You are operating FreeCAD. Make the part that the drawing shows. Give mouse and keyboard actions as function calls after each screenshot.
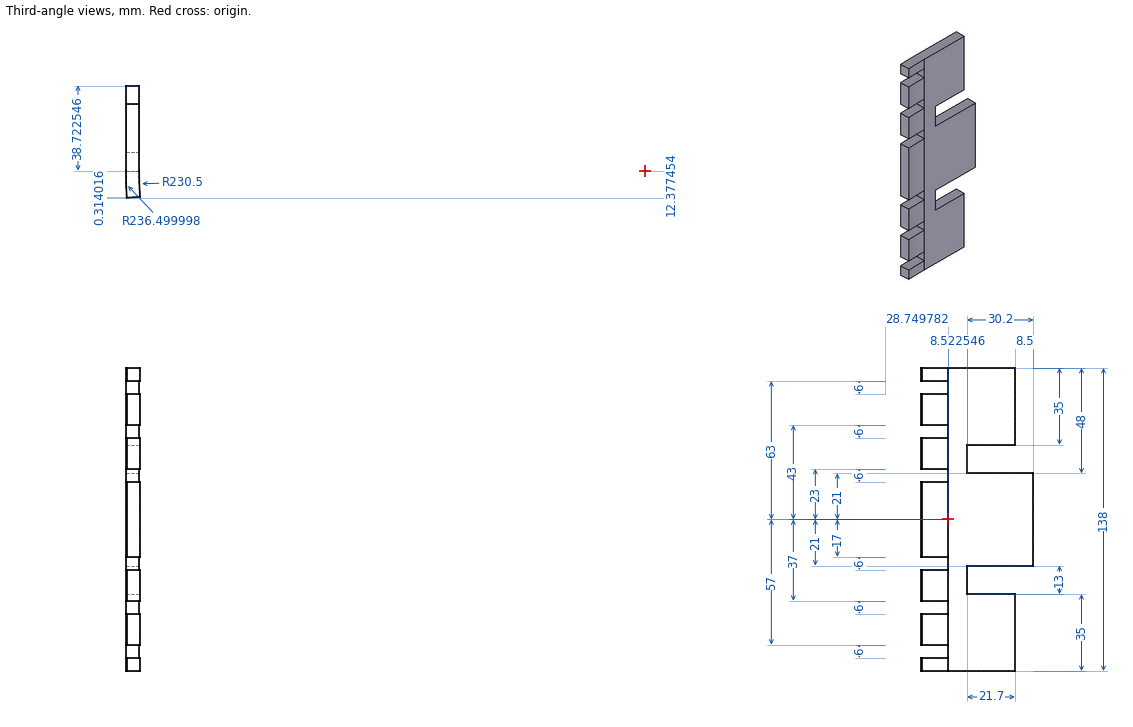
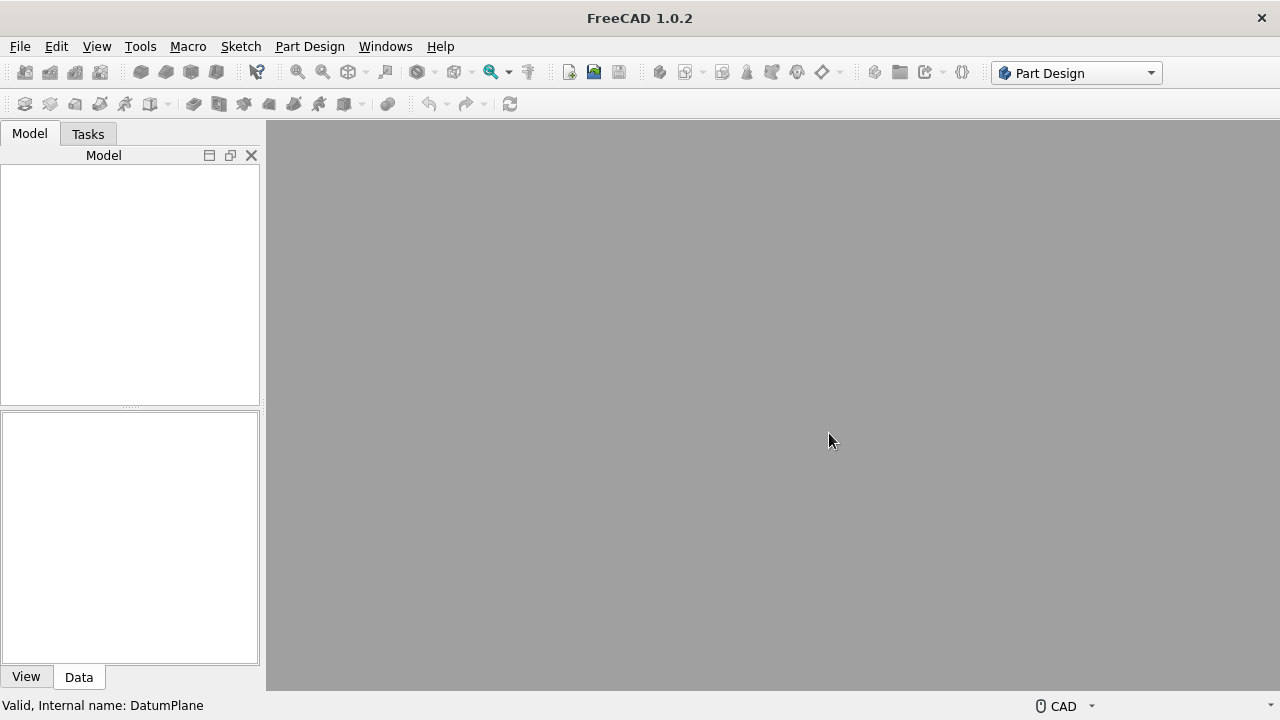
click(569, 72)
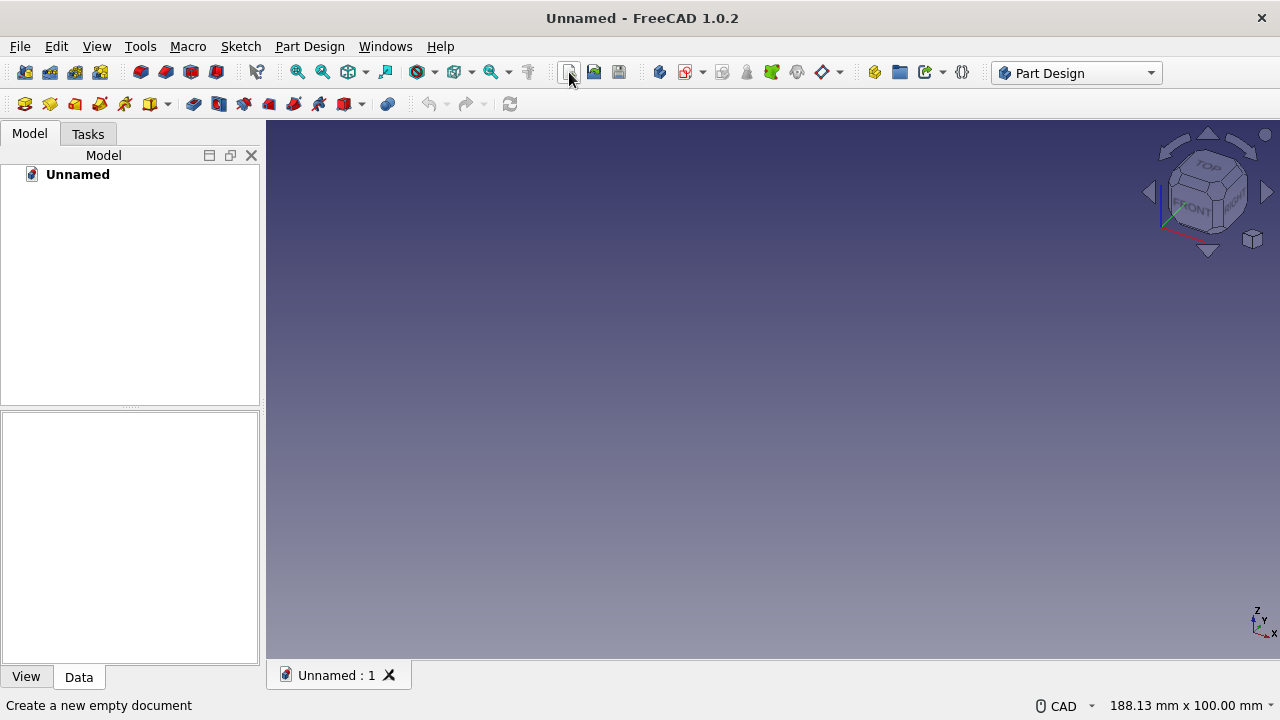
click(684, 72)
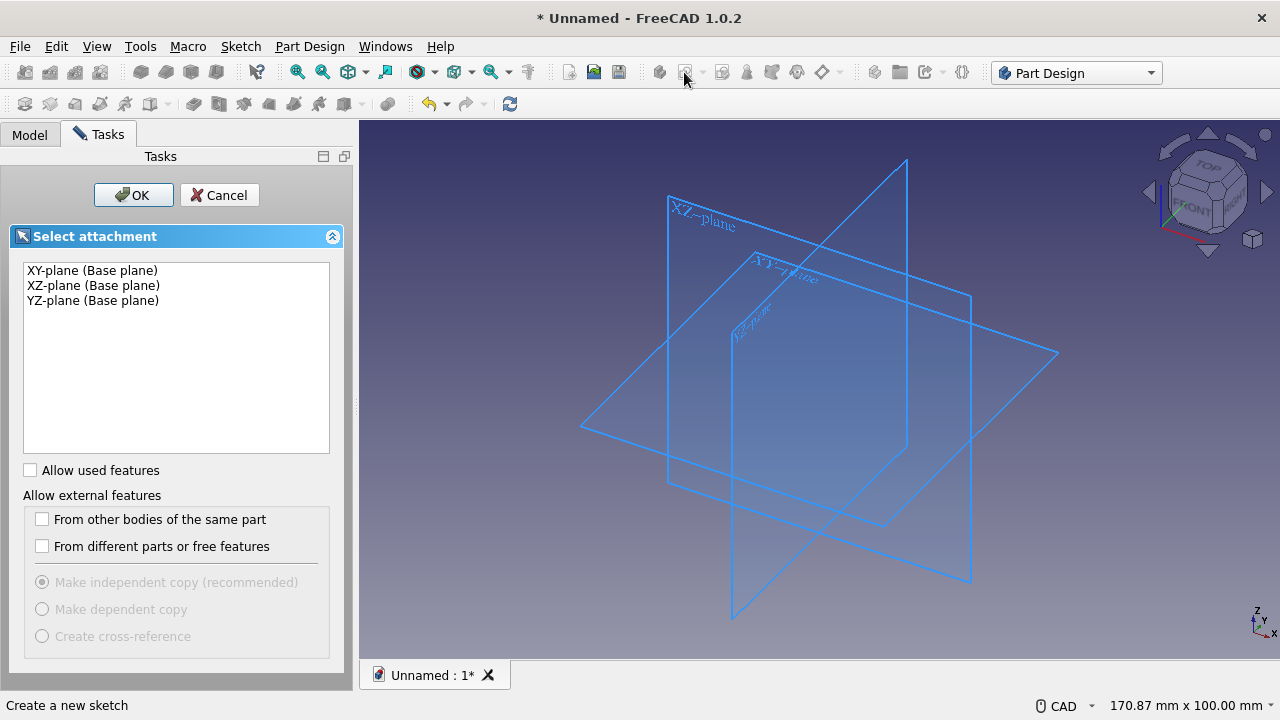
click(84, 270)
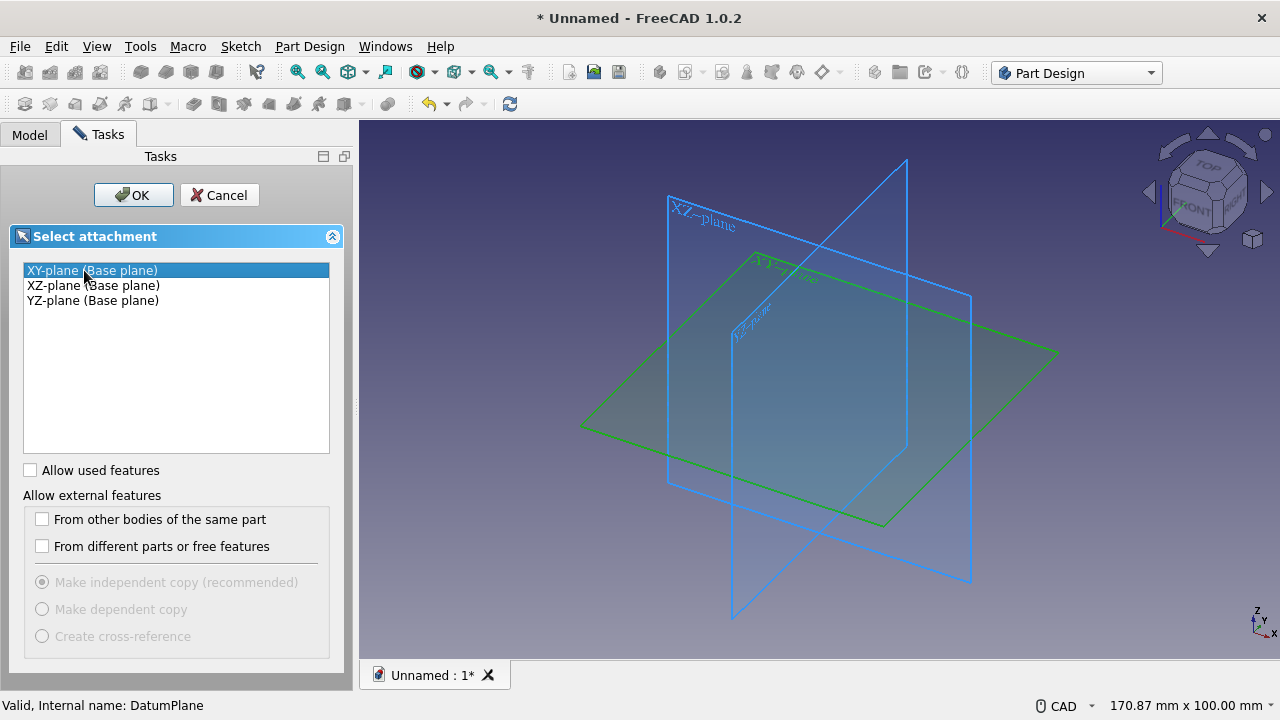
click(134, 195)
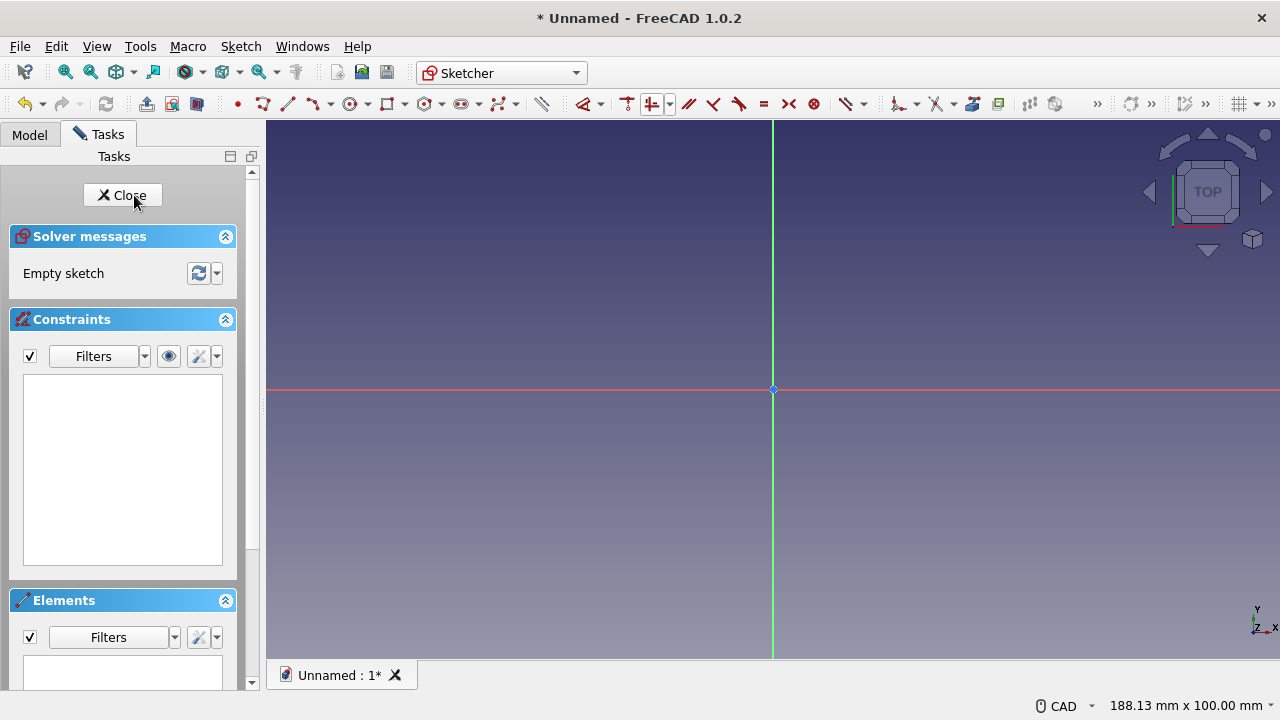
scroll(704, 390, down, 5)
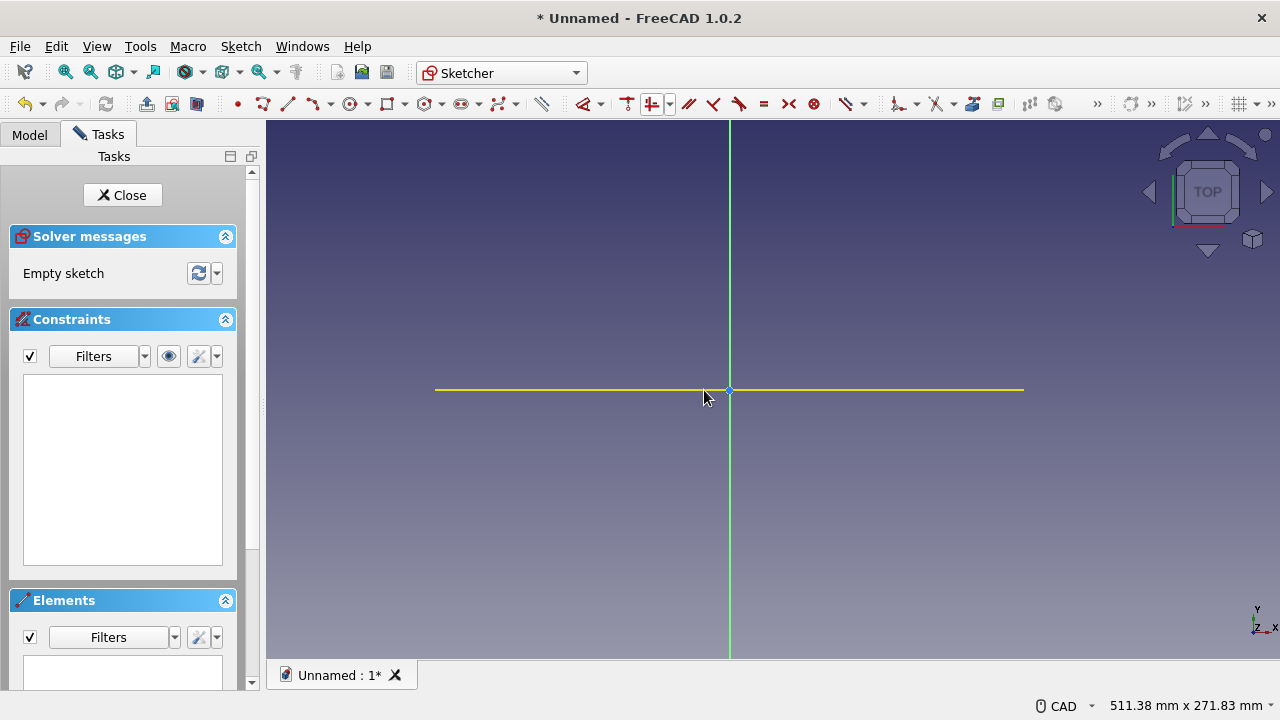
scroll(704, 390, down, 5)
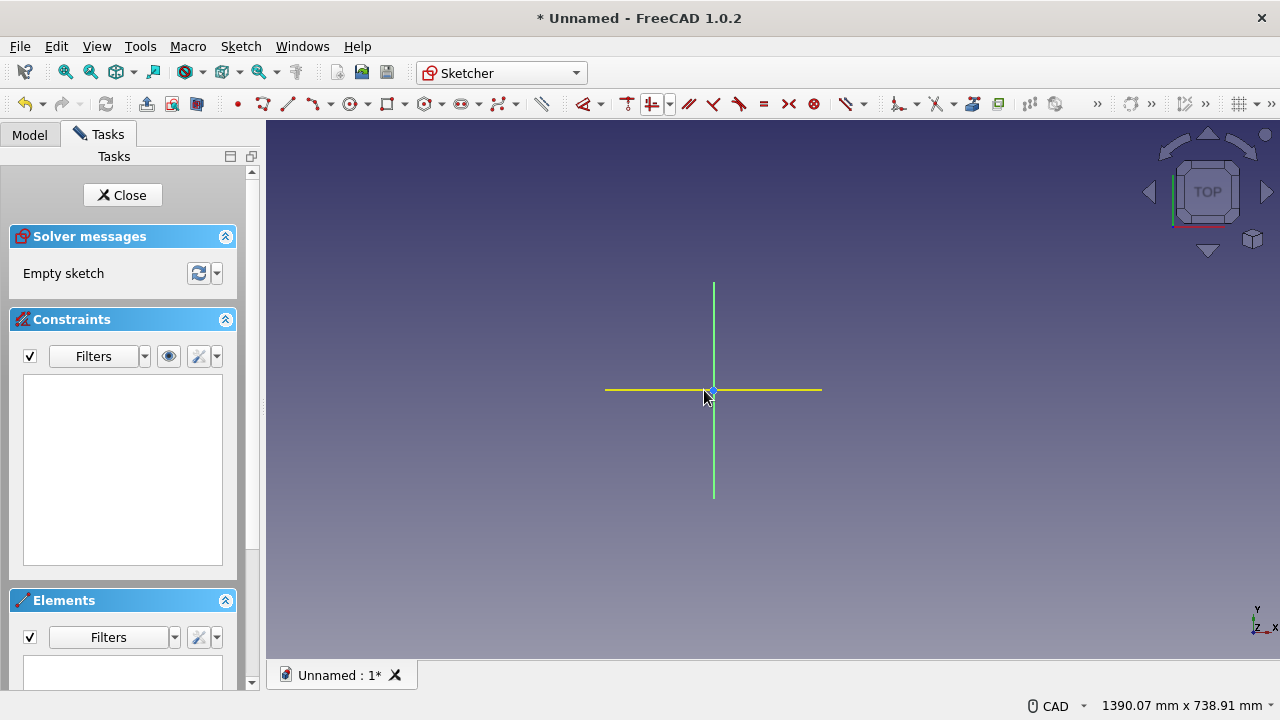
scroll(523, 380, up, 11)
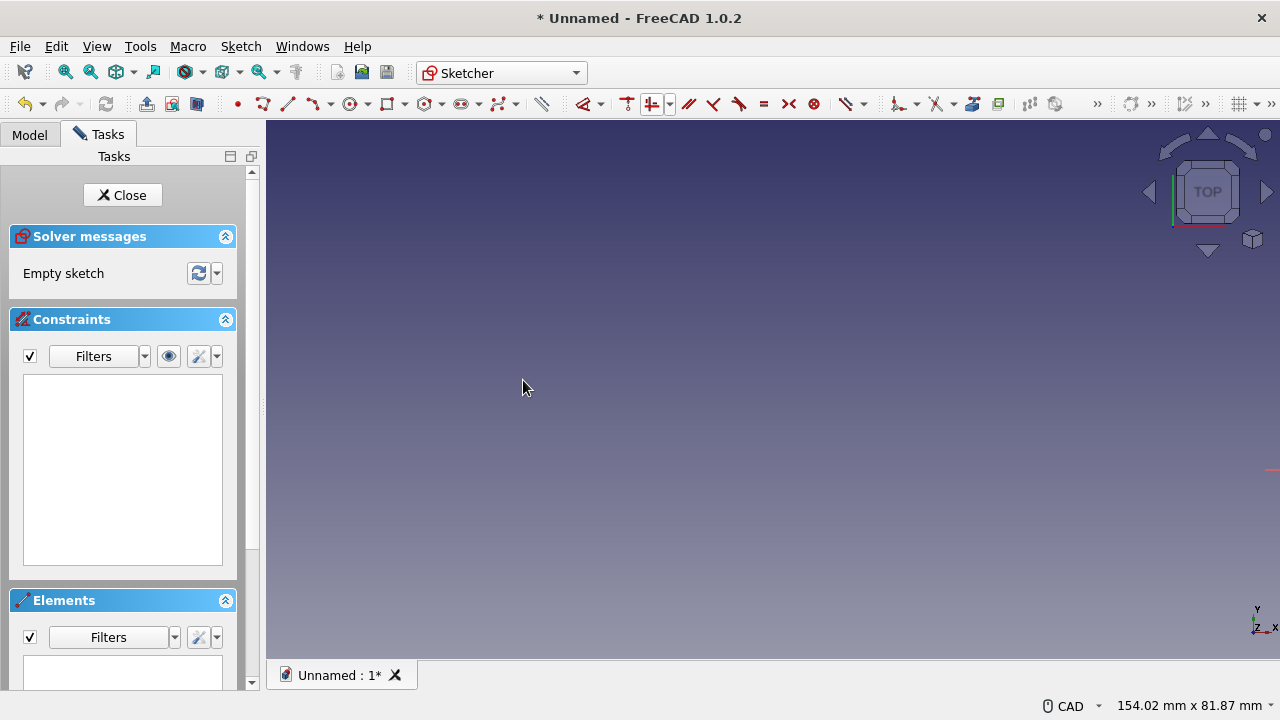
key(g)
key(l)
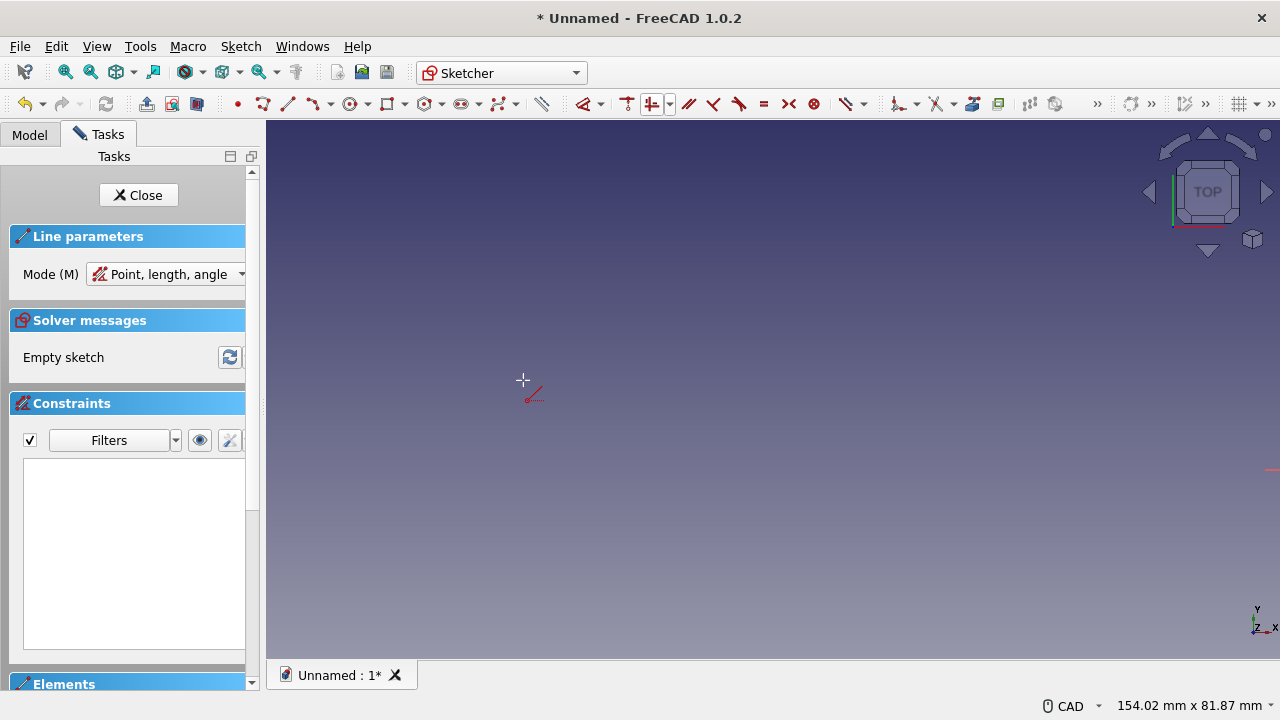
click(687, 551)
click(727, 548)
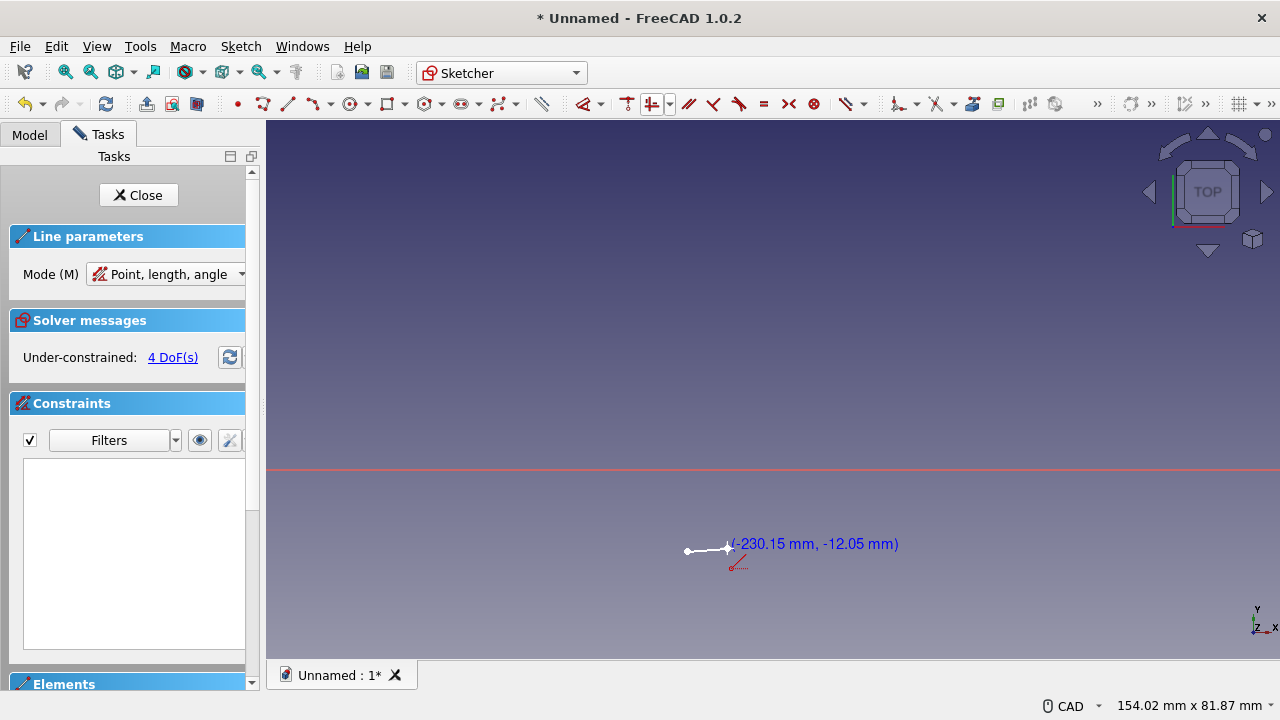
key(g)
key(m)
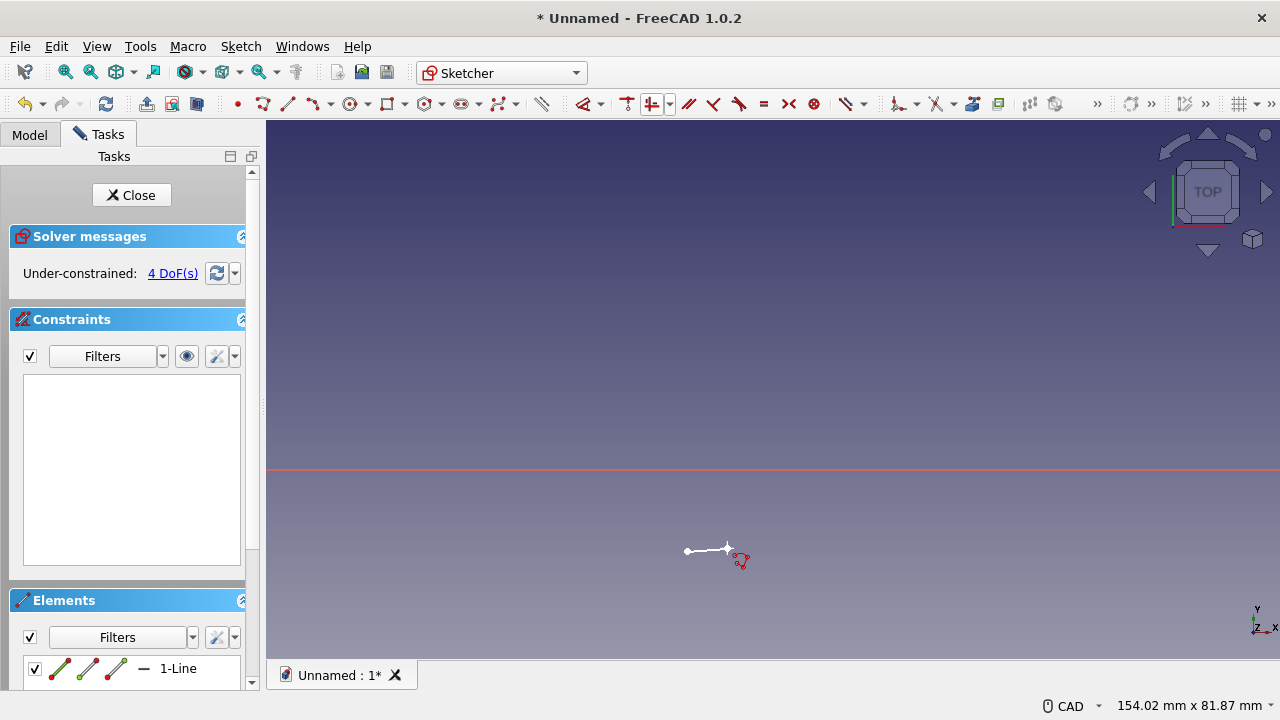
click(725, 470)
click(725, 215)
click(685, 215)
click(685, 470)
right_click(685, 470)